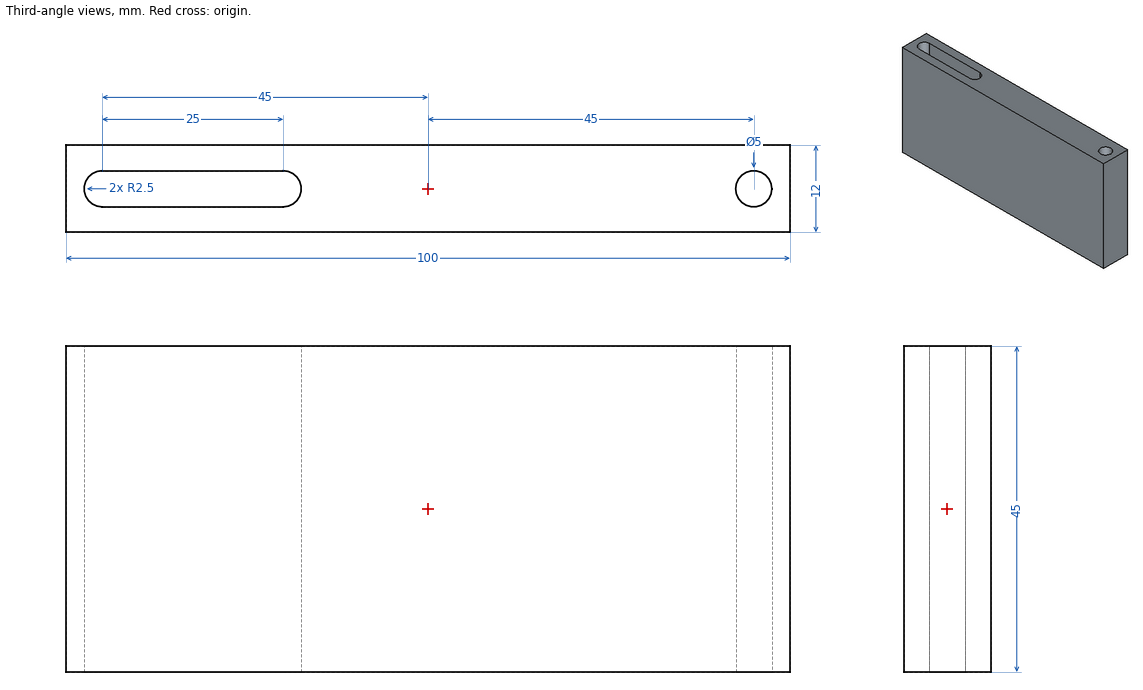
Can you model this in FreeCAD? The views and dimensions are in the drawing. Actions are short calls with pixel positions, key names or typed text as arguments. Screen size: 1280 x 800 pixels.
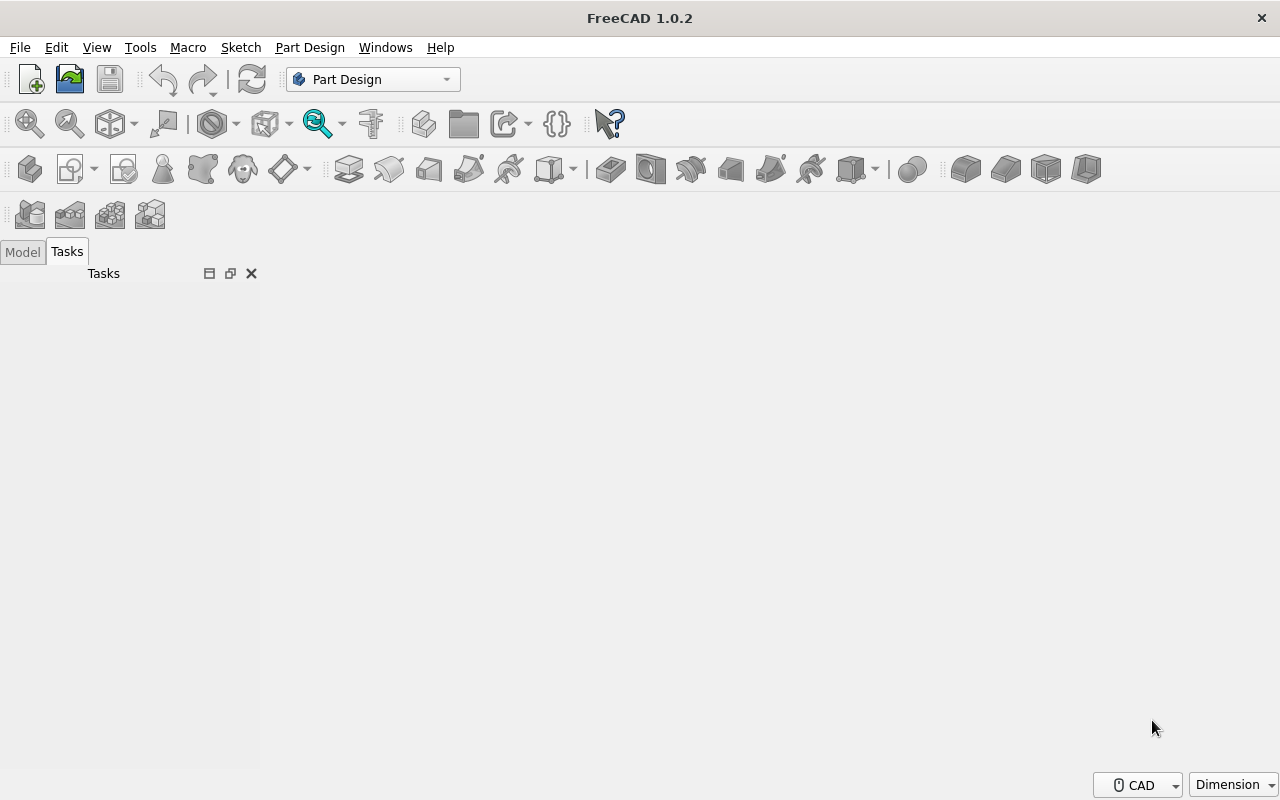
click(30, 80)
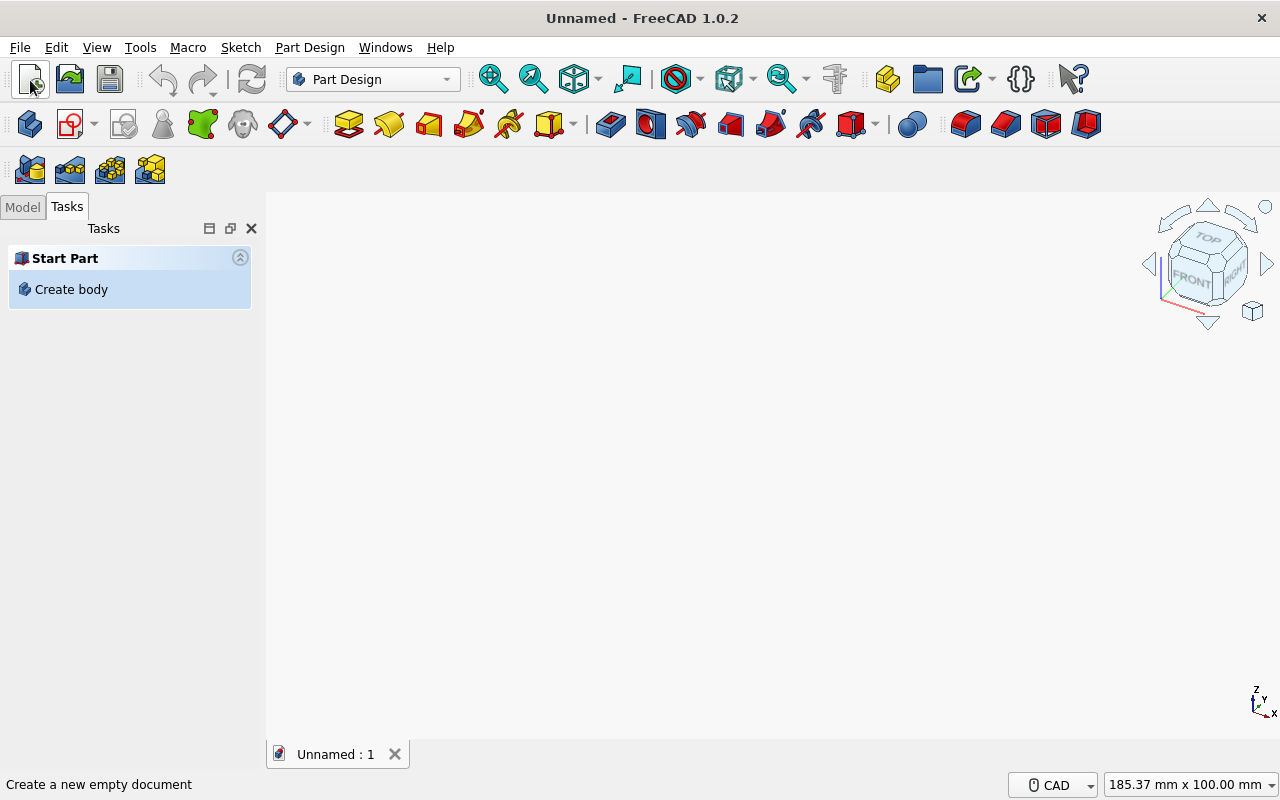
click(70, 124)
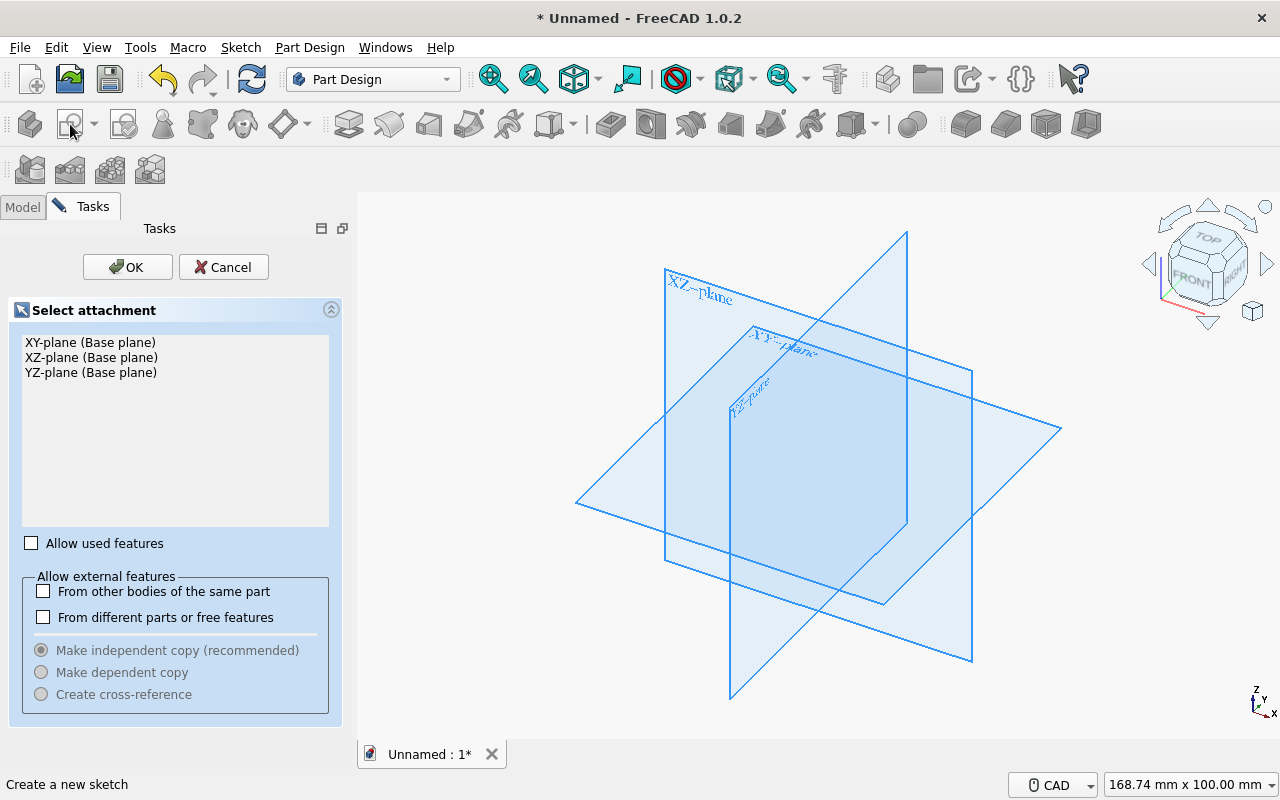
click(82, 342)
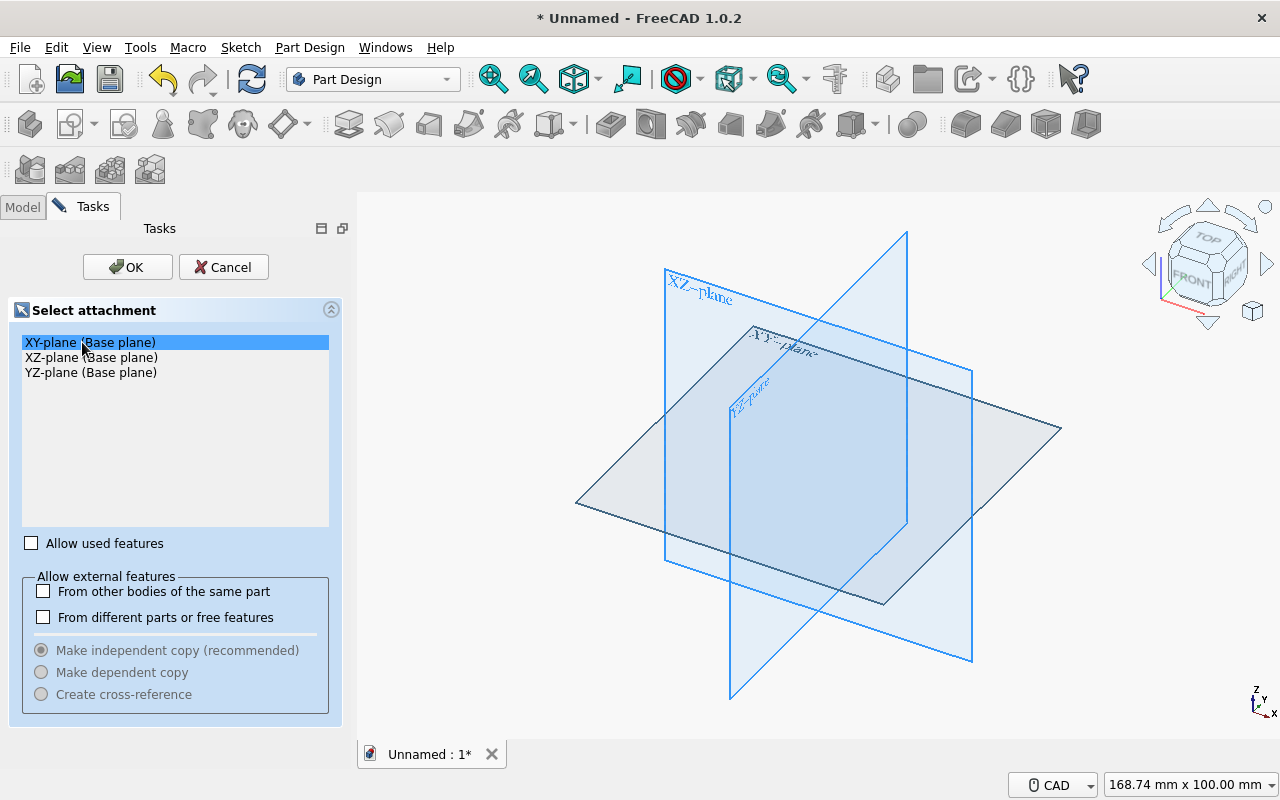
click(128, 267)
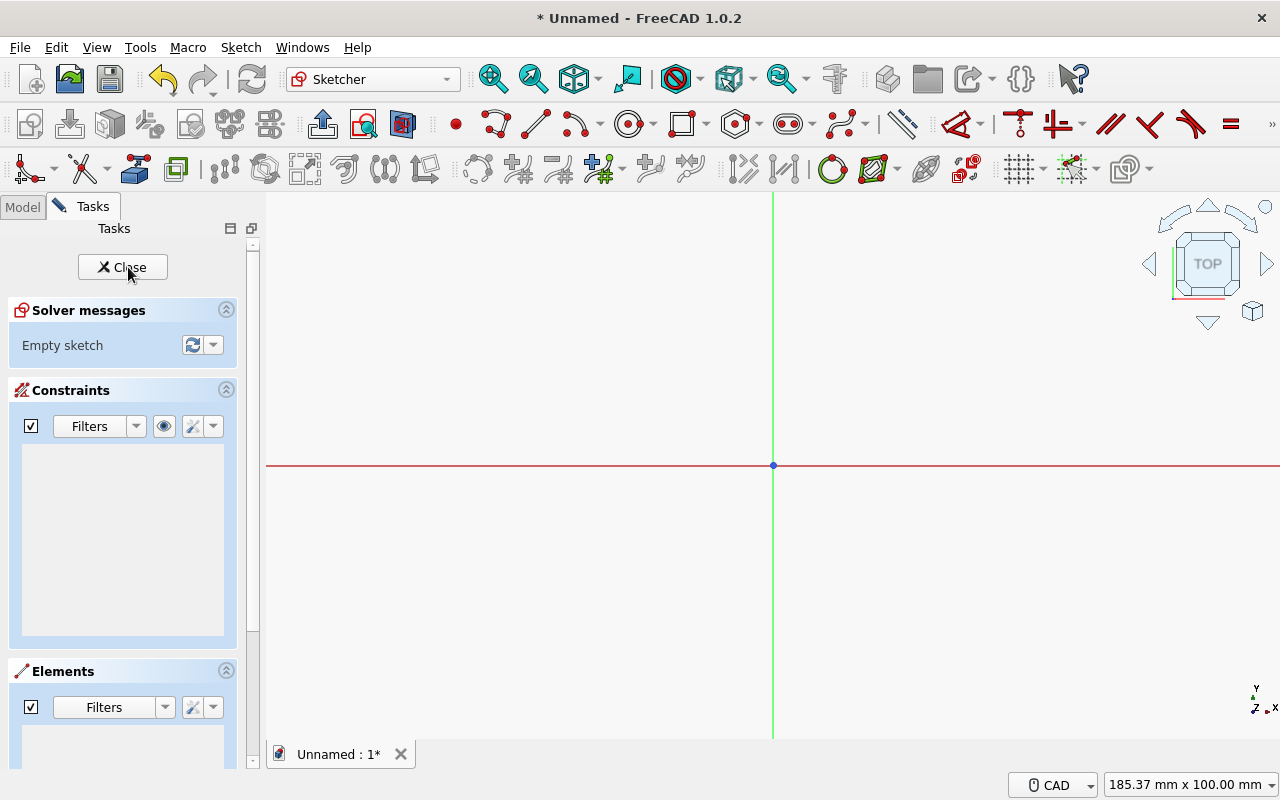
click(708, 124)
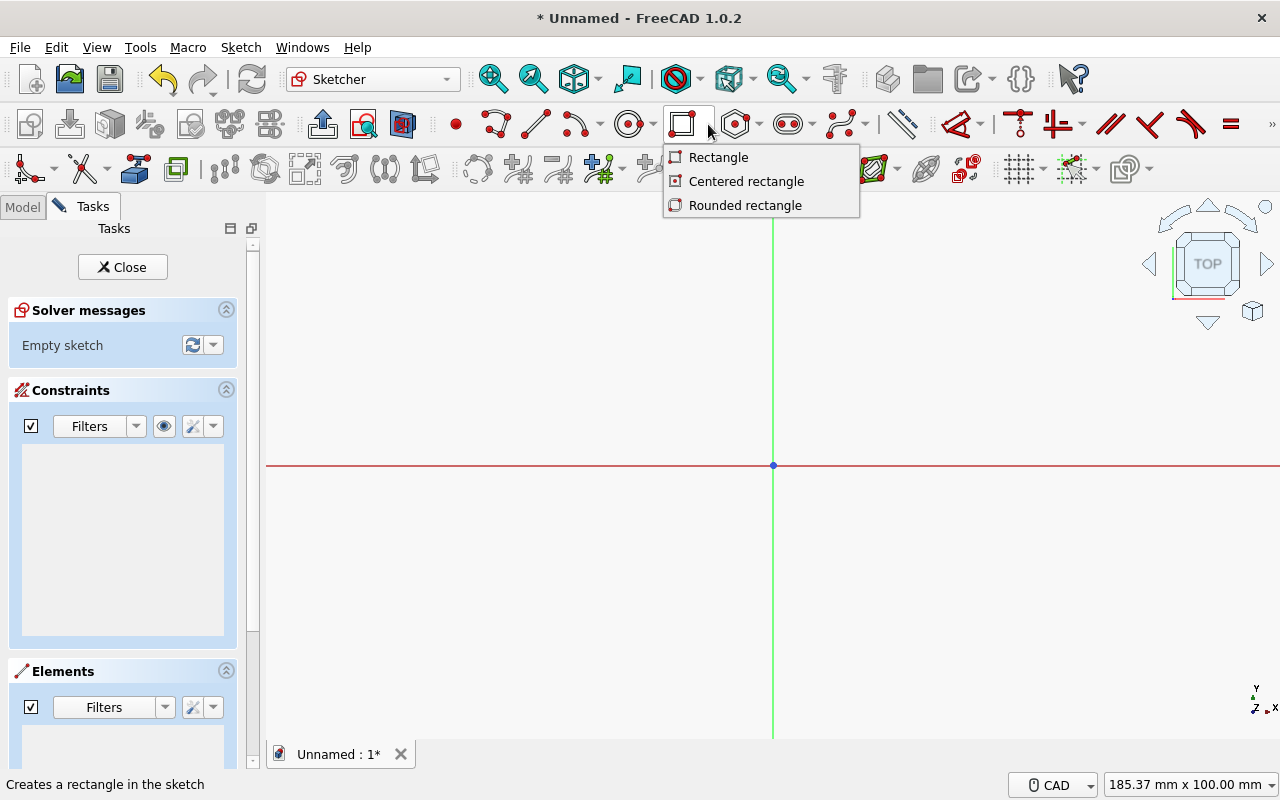
click(762, 181)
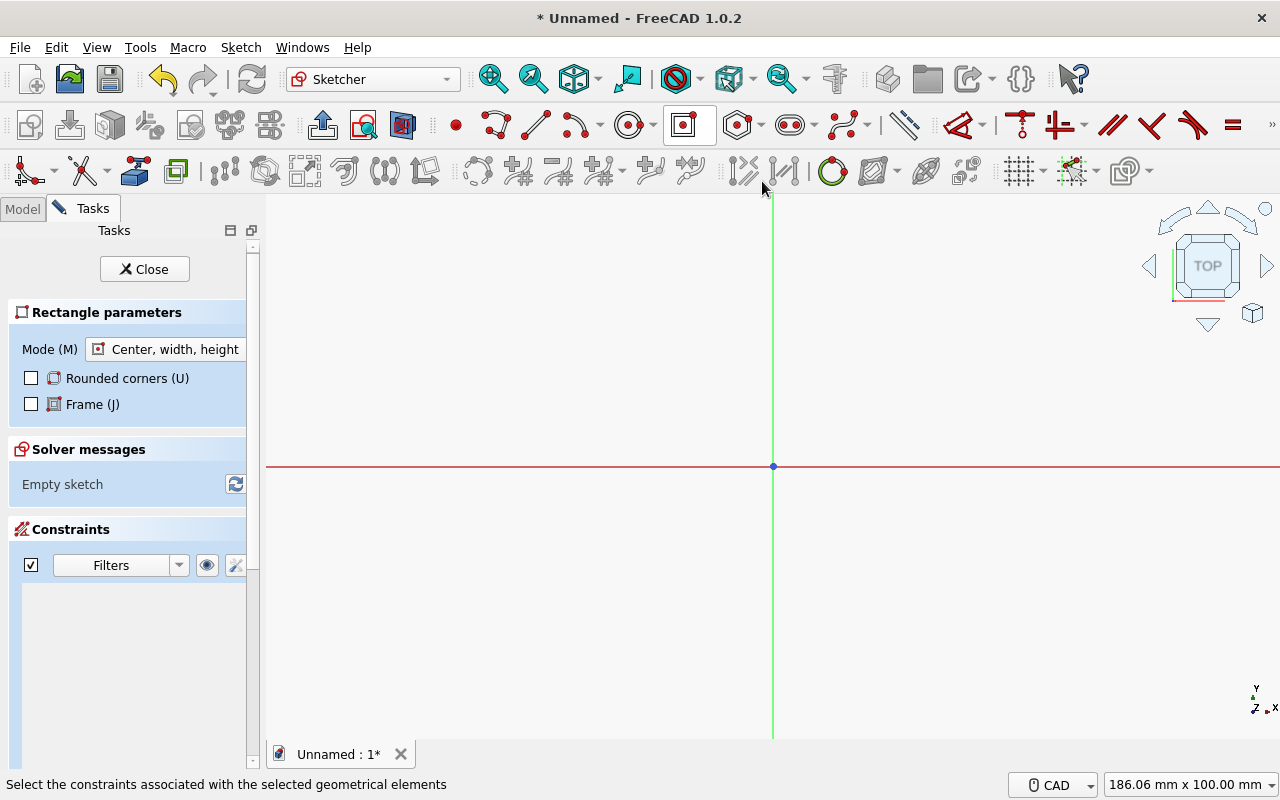
click(773, 466)
click(1046, 434)
key(Escape)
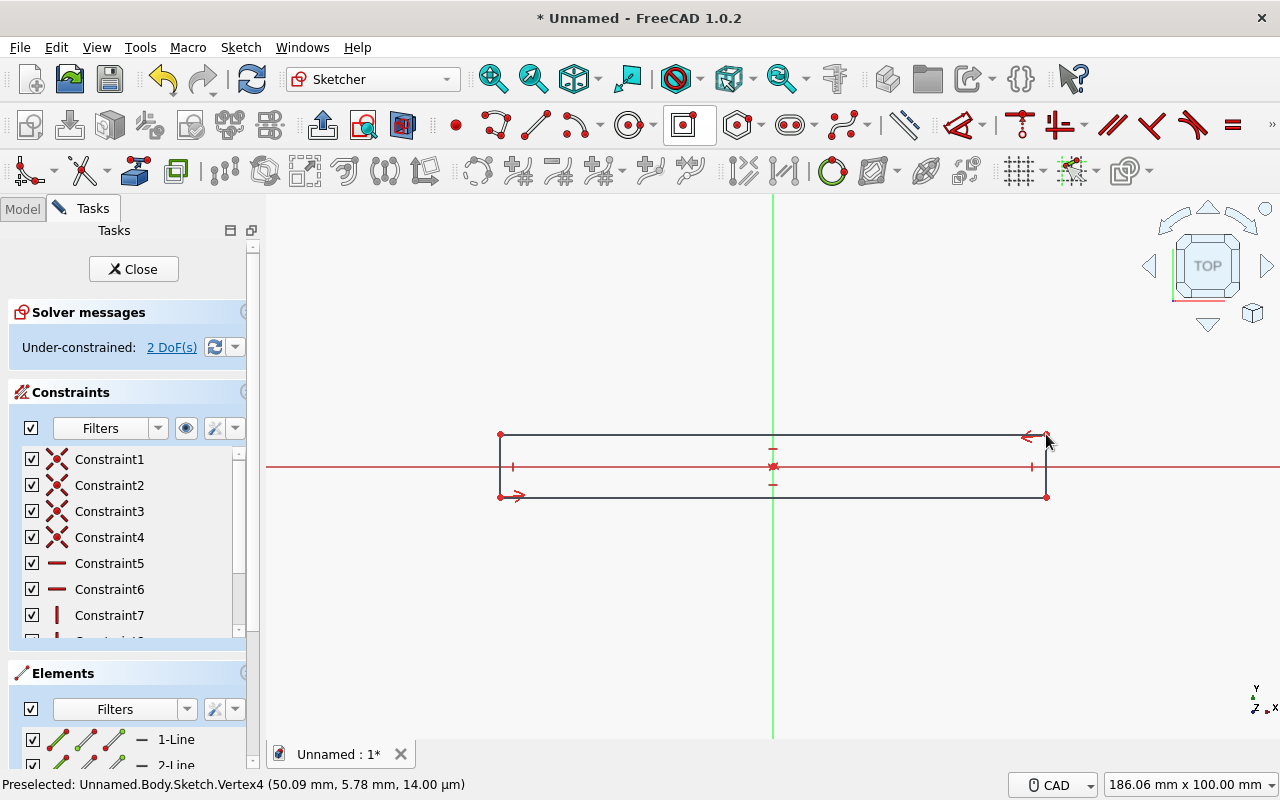
click(958, 126)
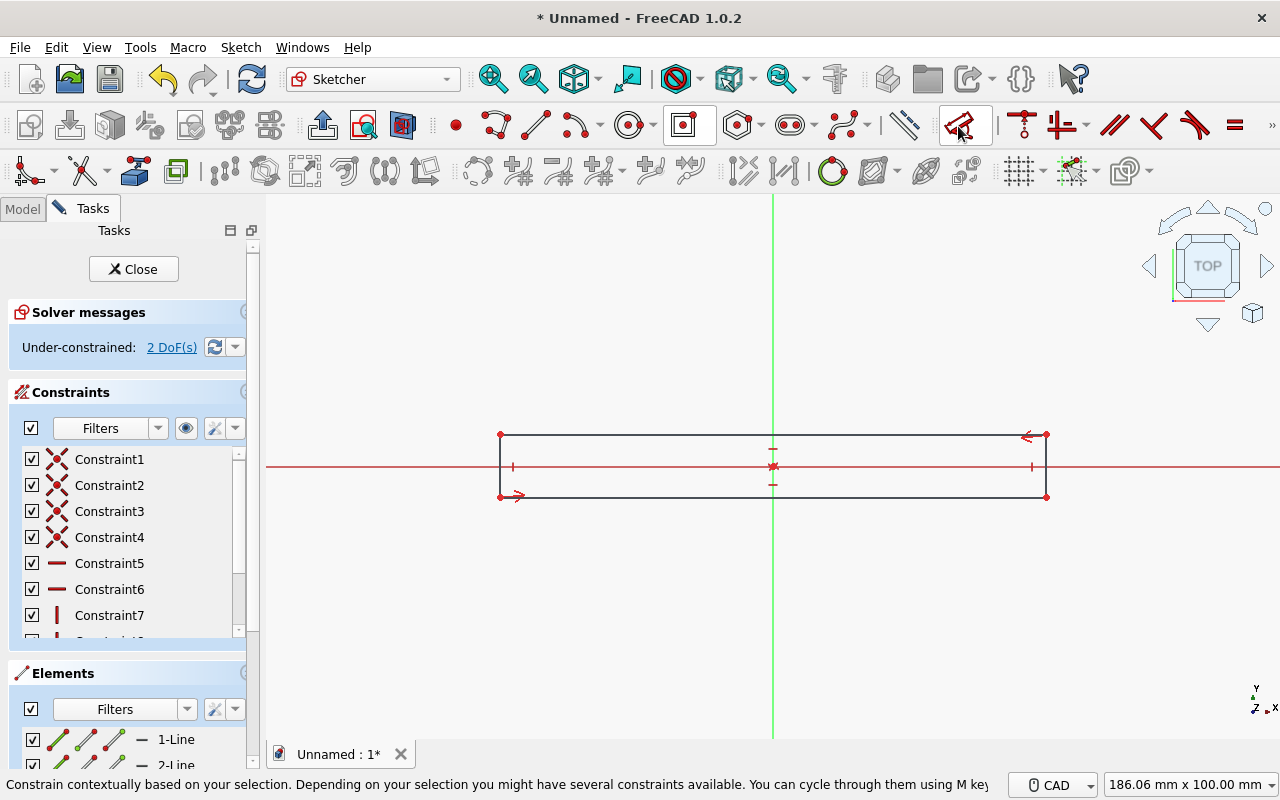
click(1046, 479)
click(1080, 452)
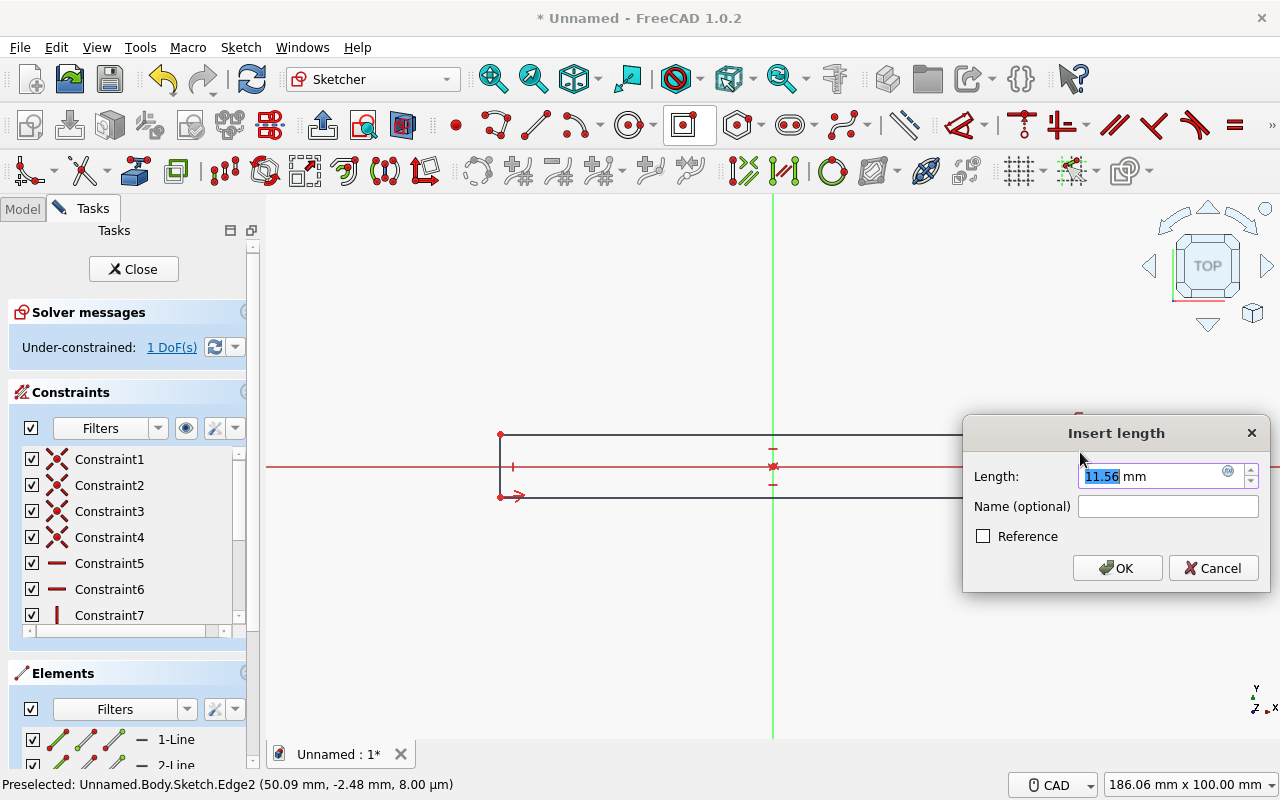
text(12)
key(Return)